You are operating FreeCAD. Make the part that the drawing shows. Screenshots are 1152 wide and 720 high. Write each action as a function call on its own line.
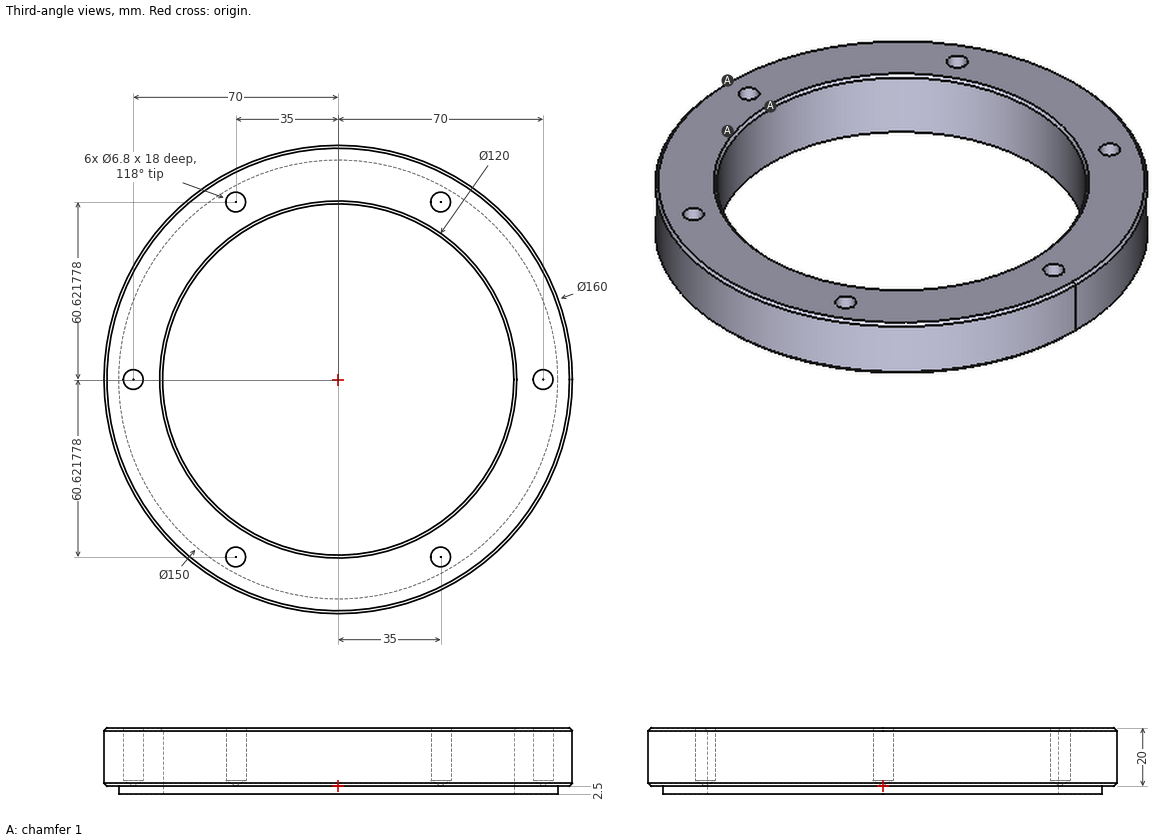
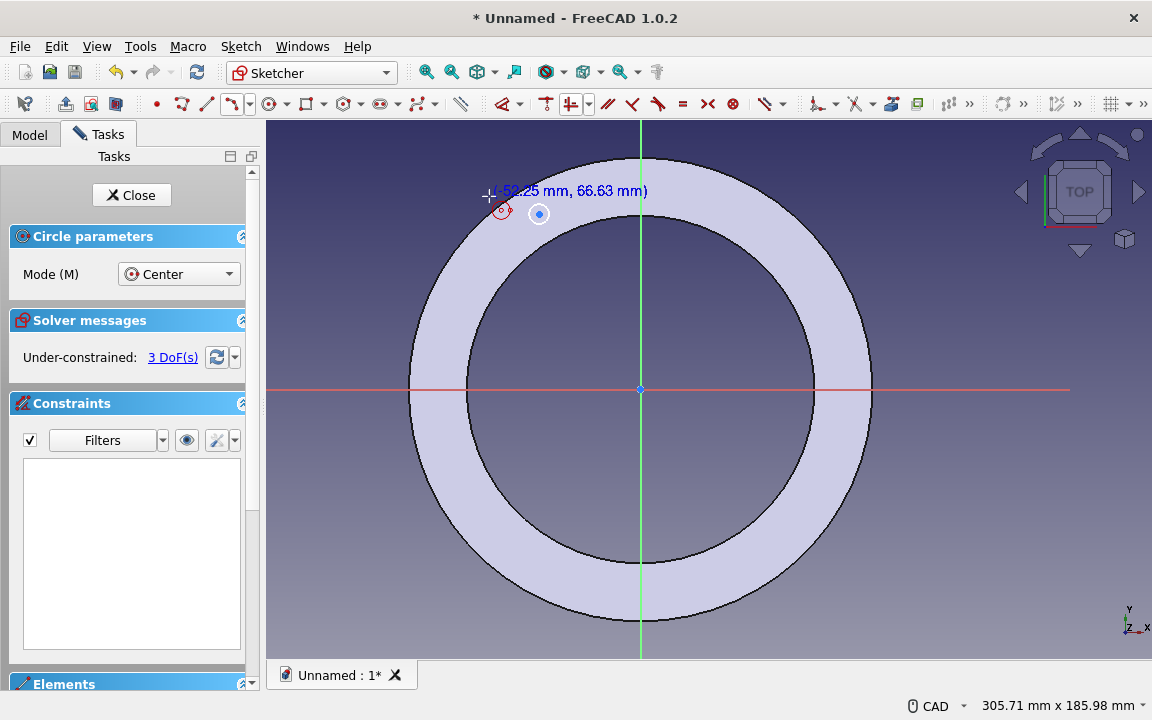
scroll(438, 390, up, 5)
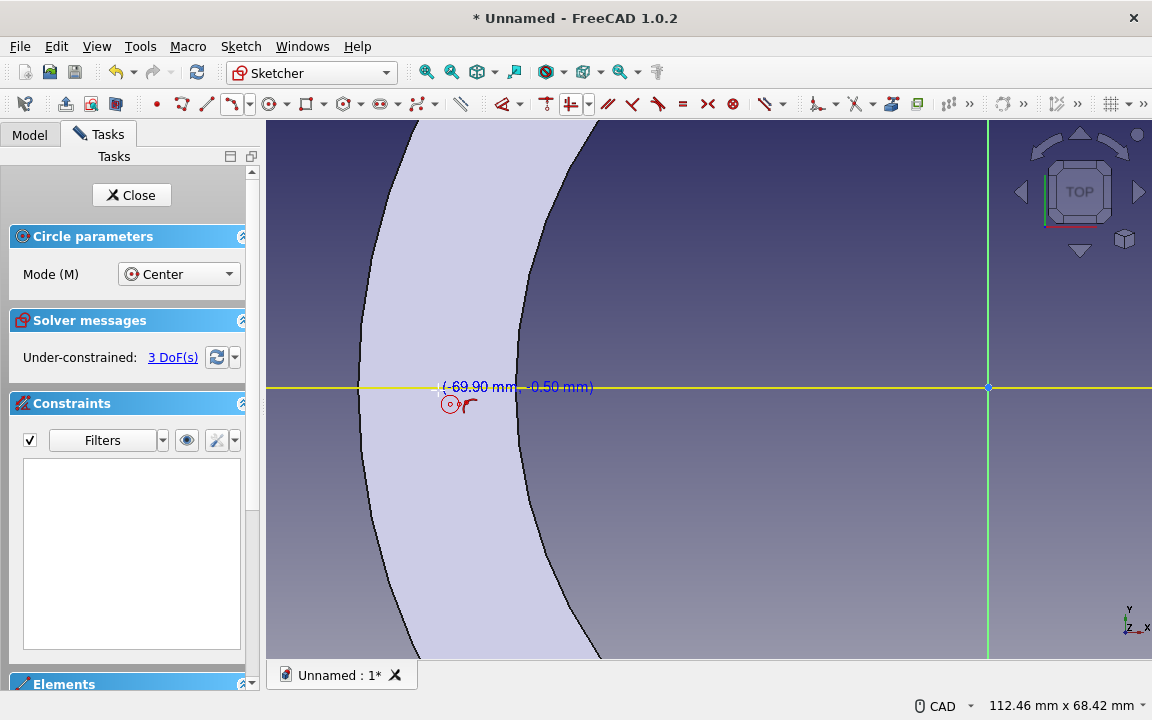
click(437, 388)
click(456, 369)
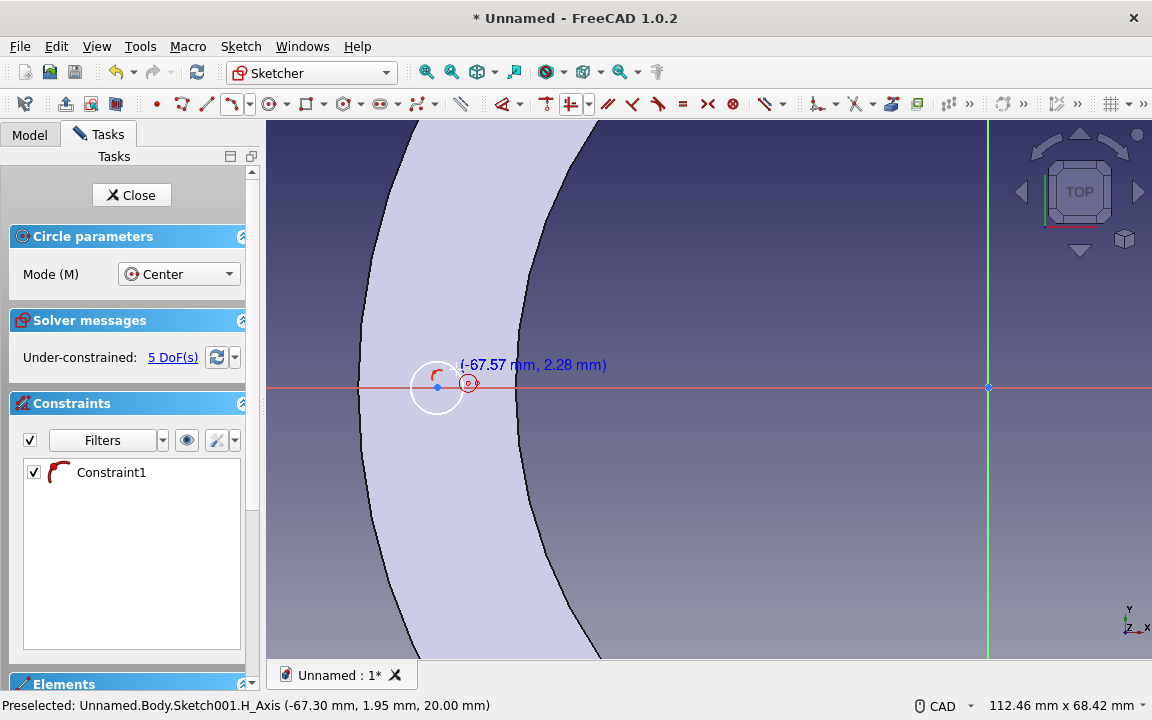
scroll(438, 390, down, 5)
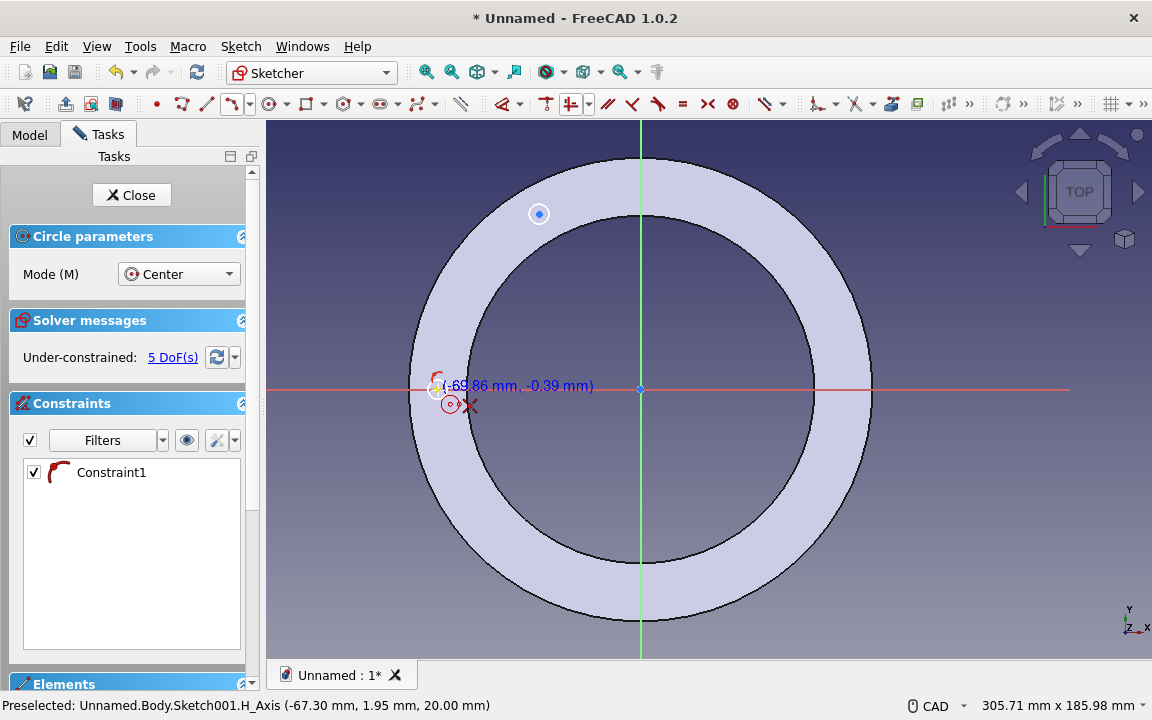
scroll(539, 565, up, 5)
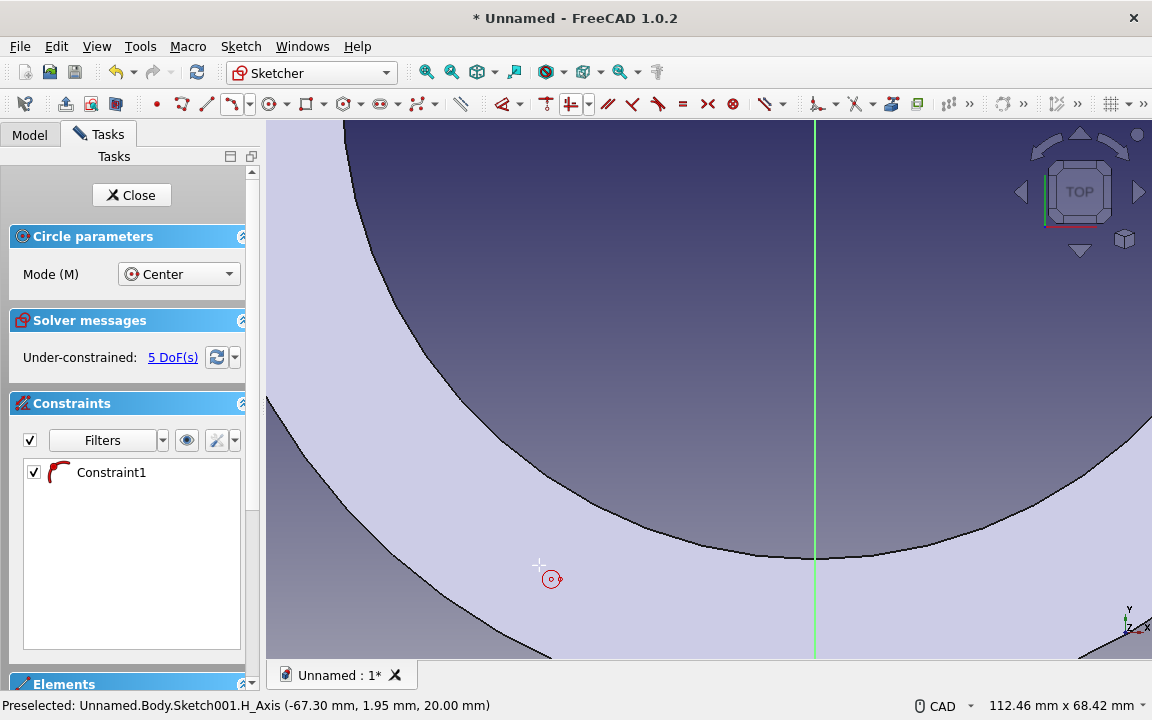
click(539, 564)
click(558, 545)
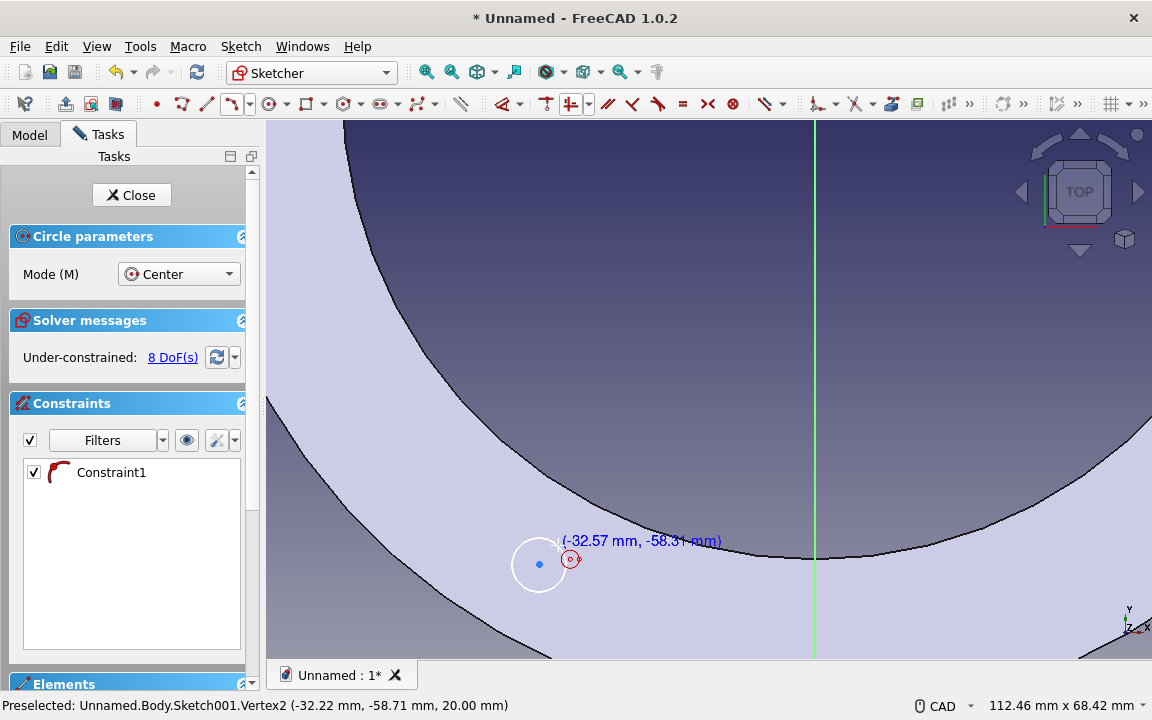
scroll(539, 566, down, 5)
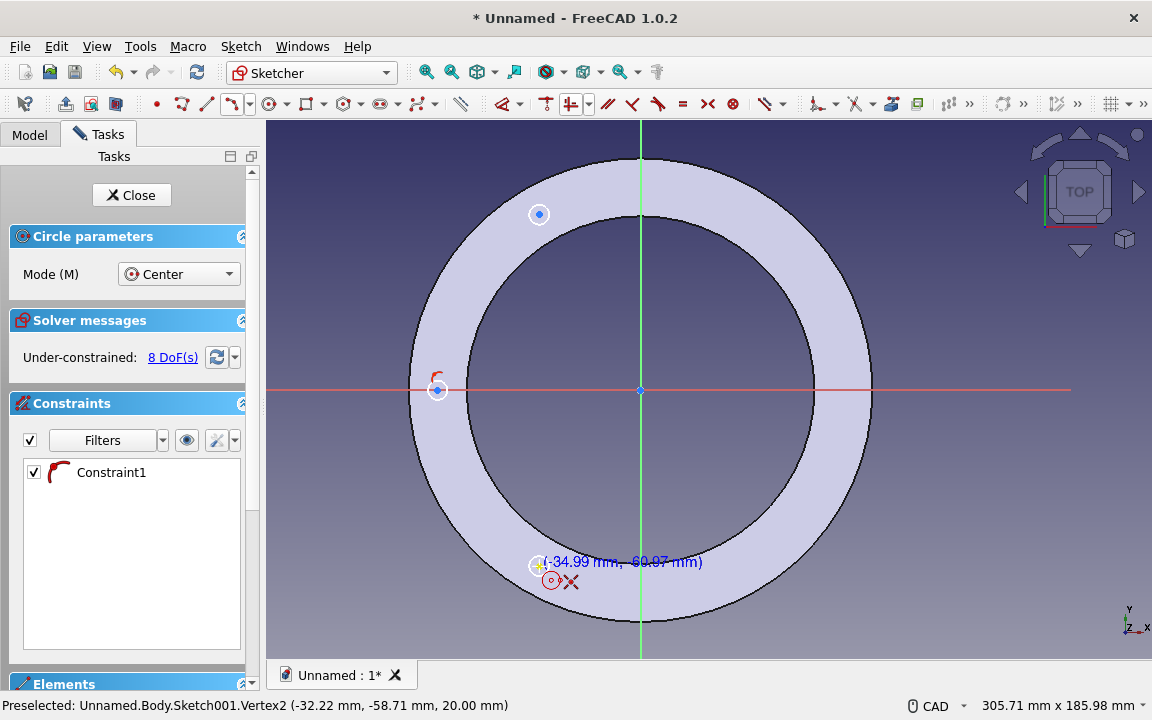
scroll(742, 566, up, 5)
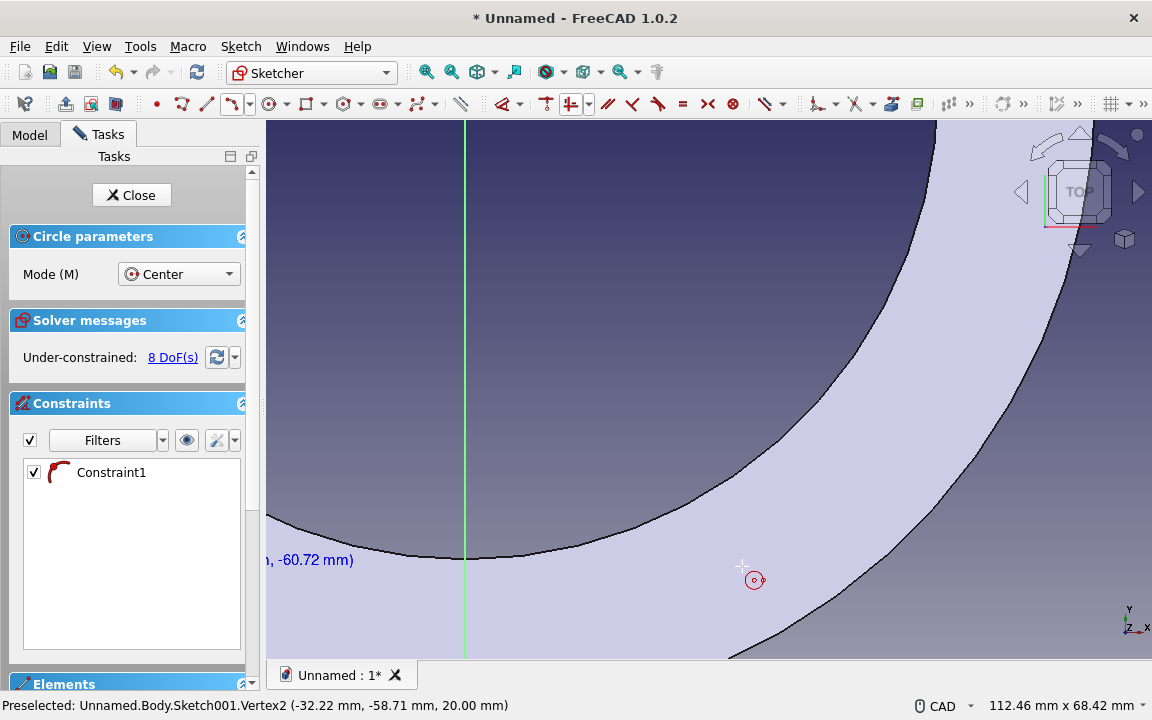
click(741, 564)
click(760, 545)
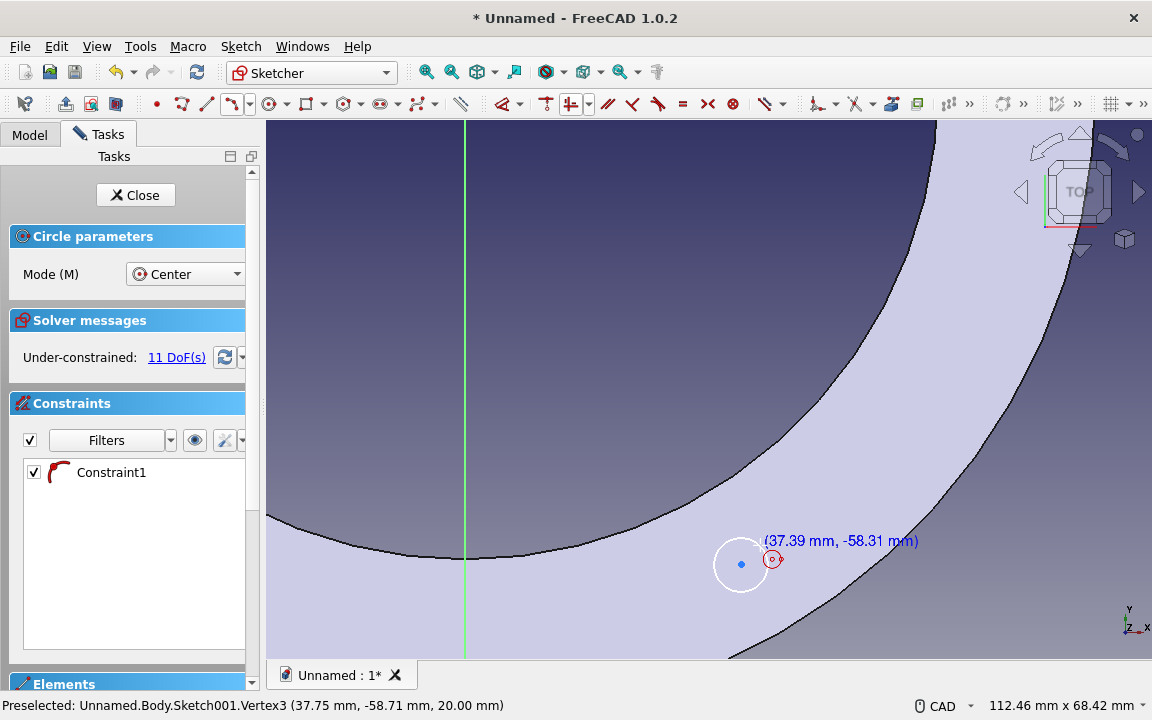
scroll(742, 566, down, 5)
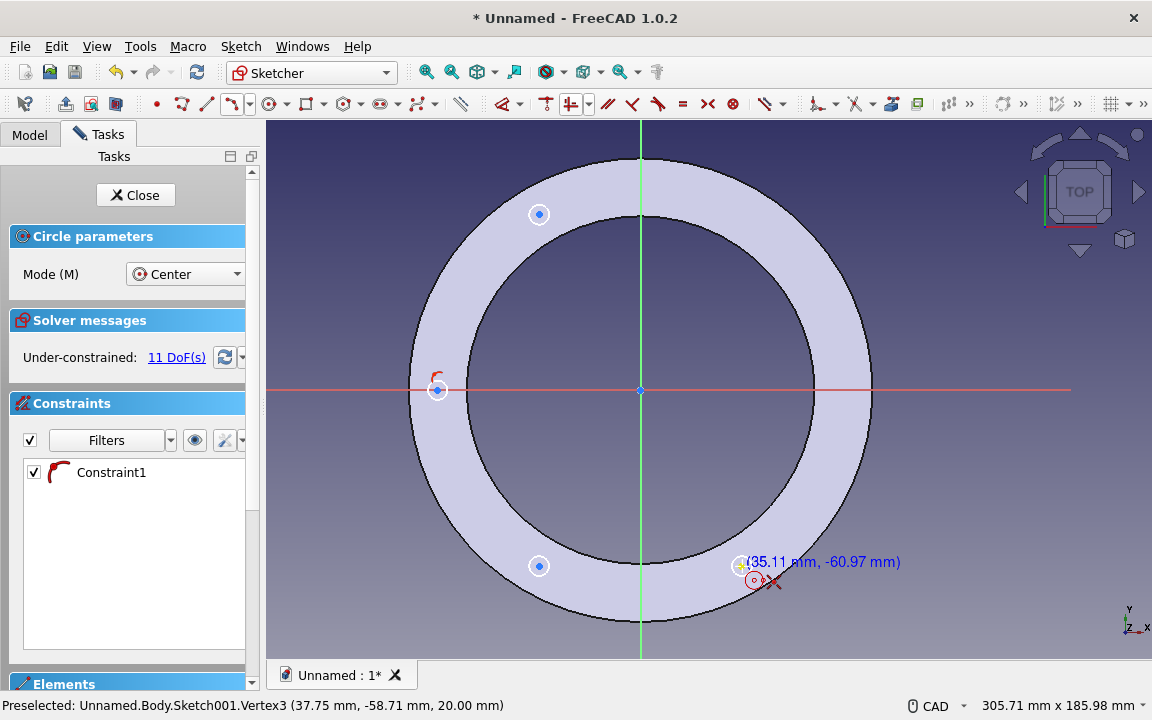
scroll(843, 390, up, 5)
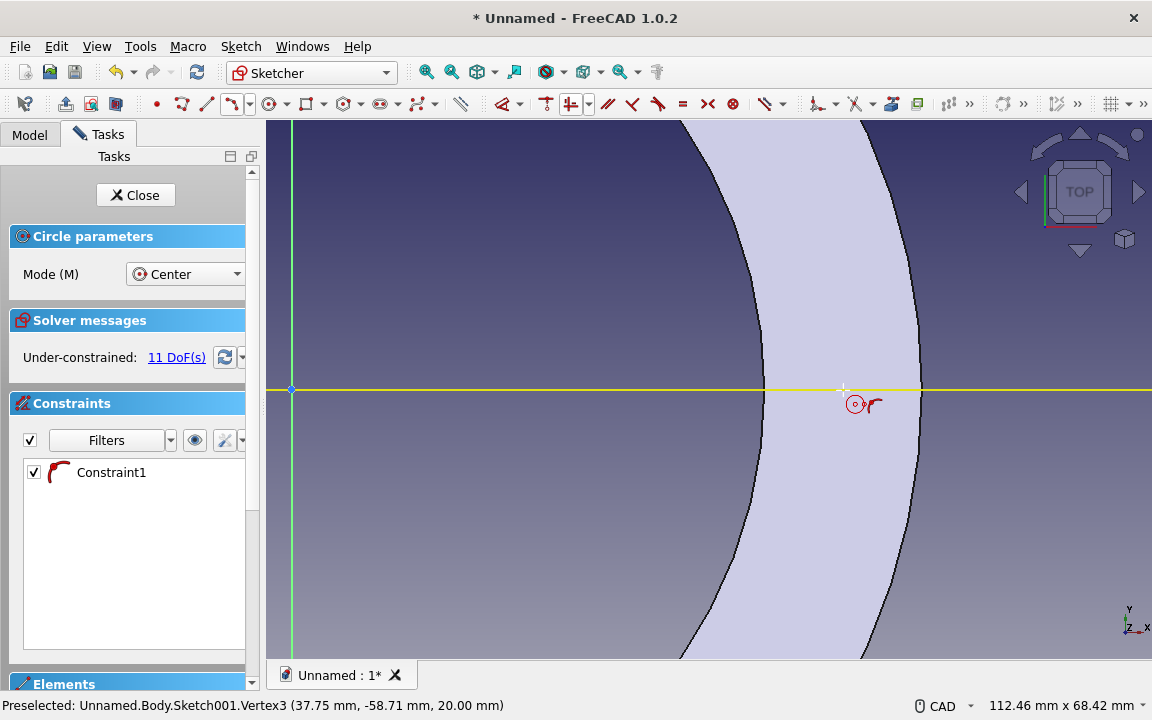
click(843, 390)
click(862, 371)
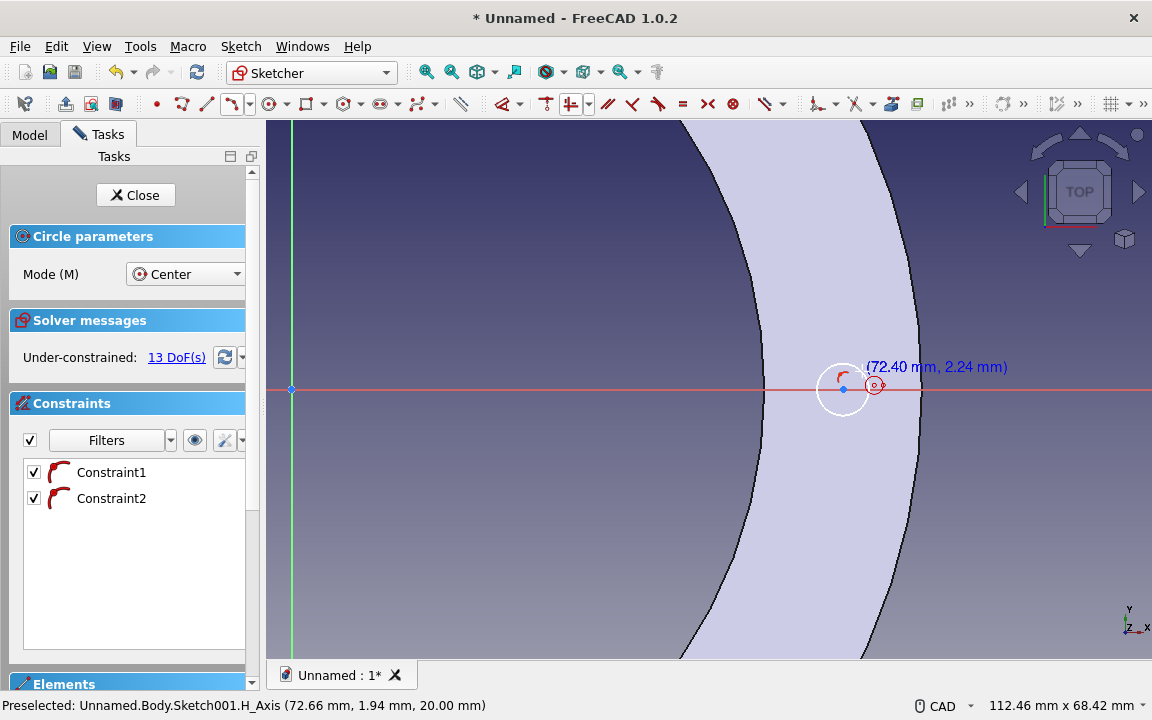
scroll(844, 389, down, 5)